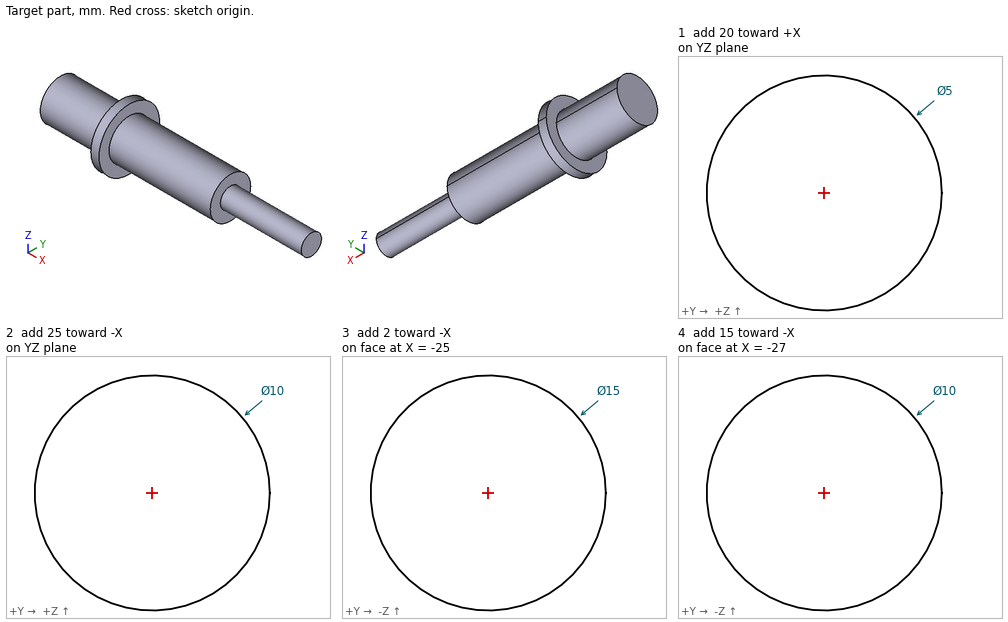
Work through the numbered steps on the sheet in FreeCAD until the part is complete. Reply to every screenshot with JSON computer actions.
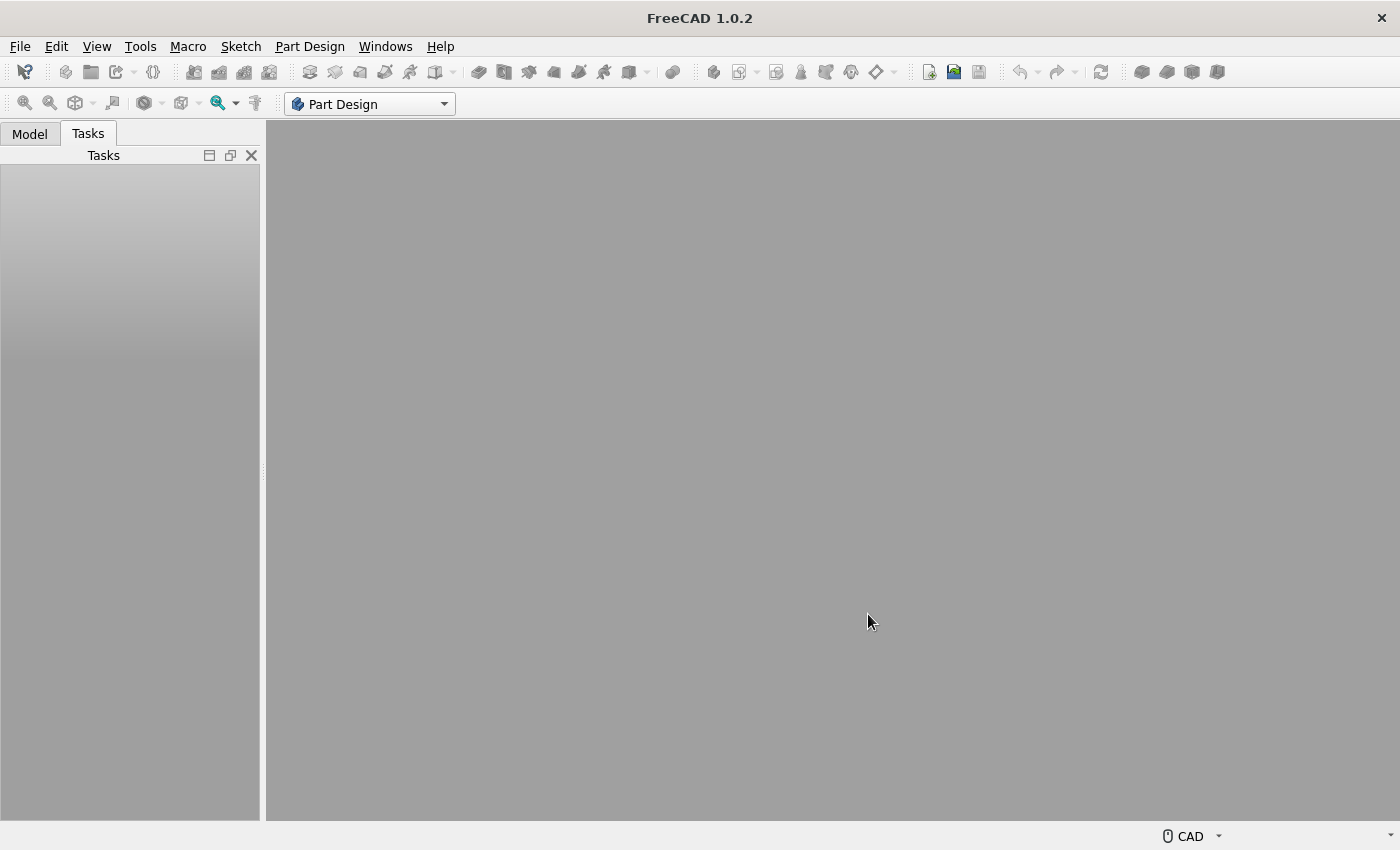
{"action": "key", "text": "ctrl+n"}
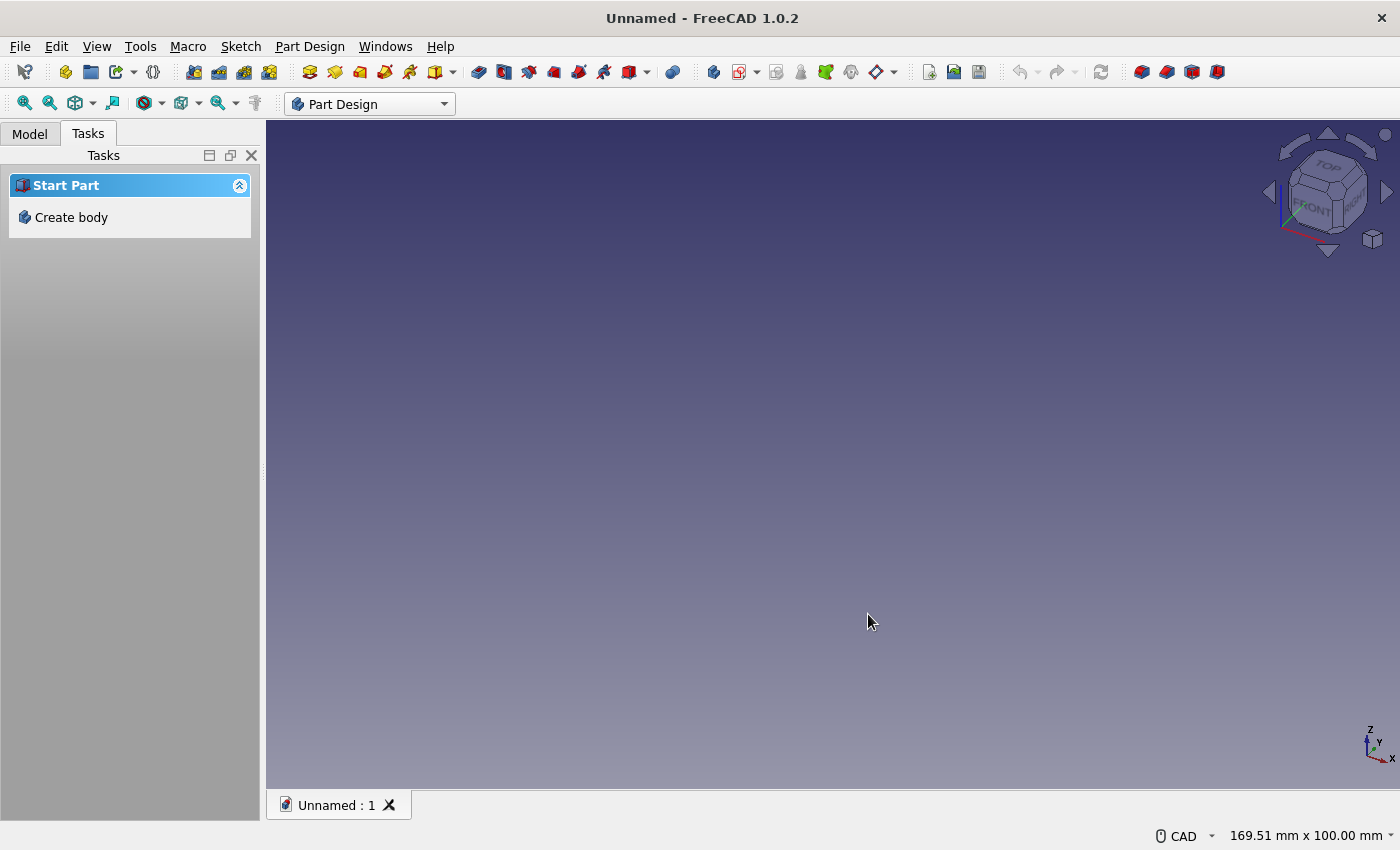
{"action": "left_click", "coordinate": [738, 72]}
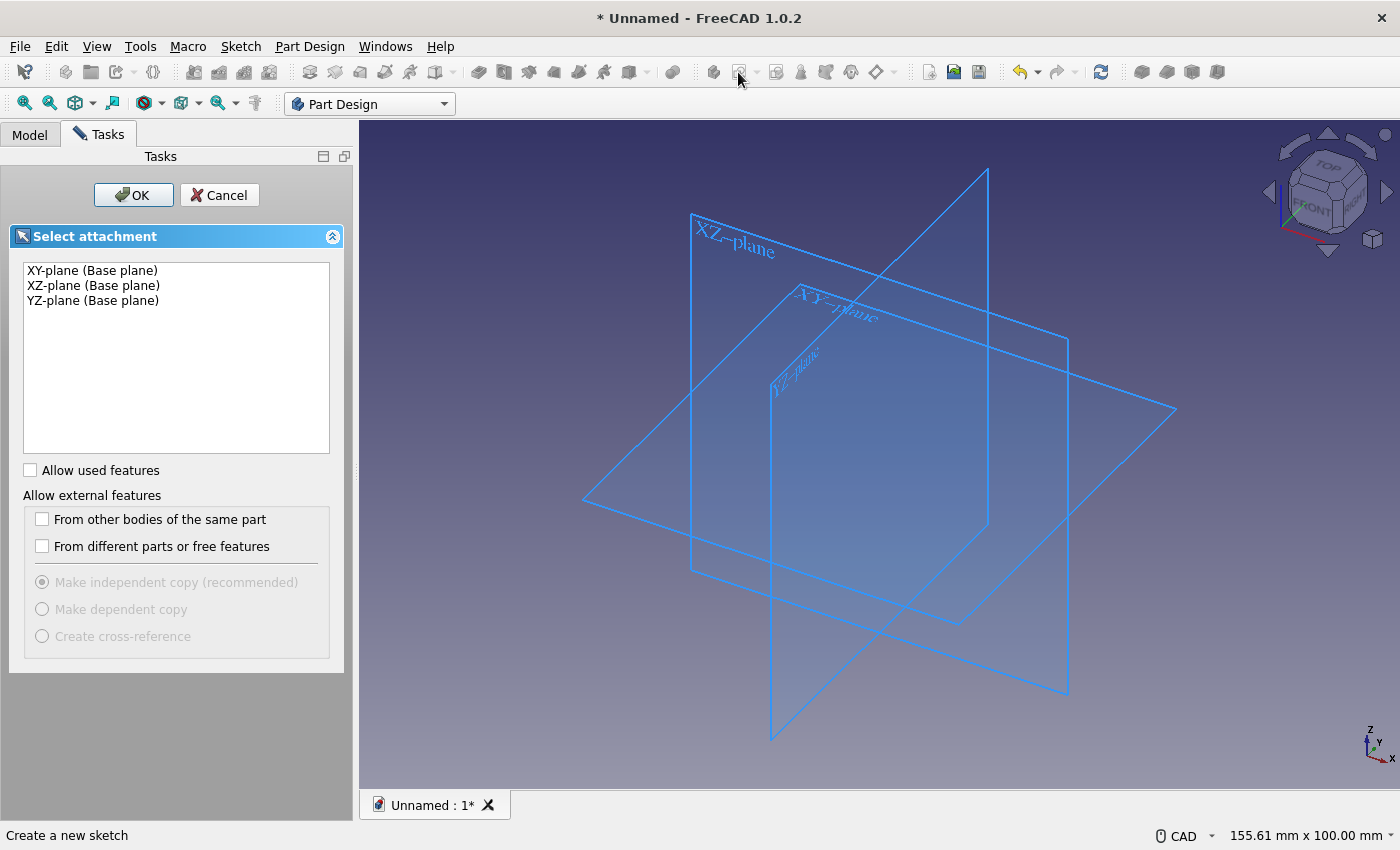
{"action": "left_click", "coordinate": [84, 300]}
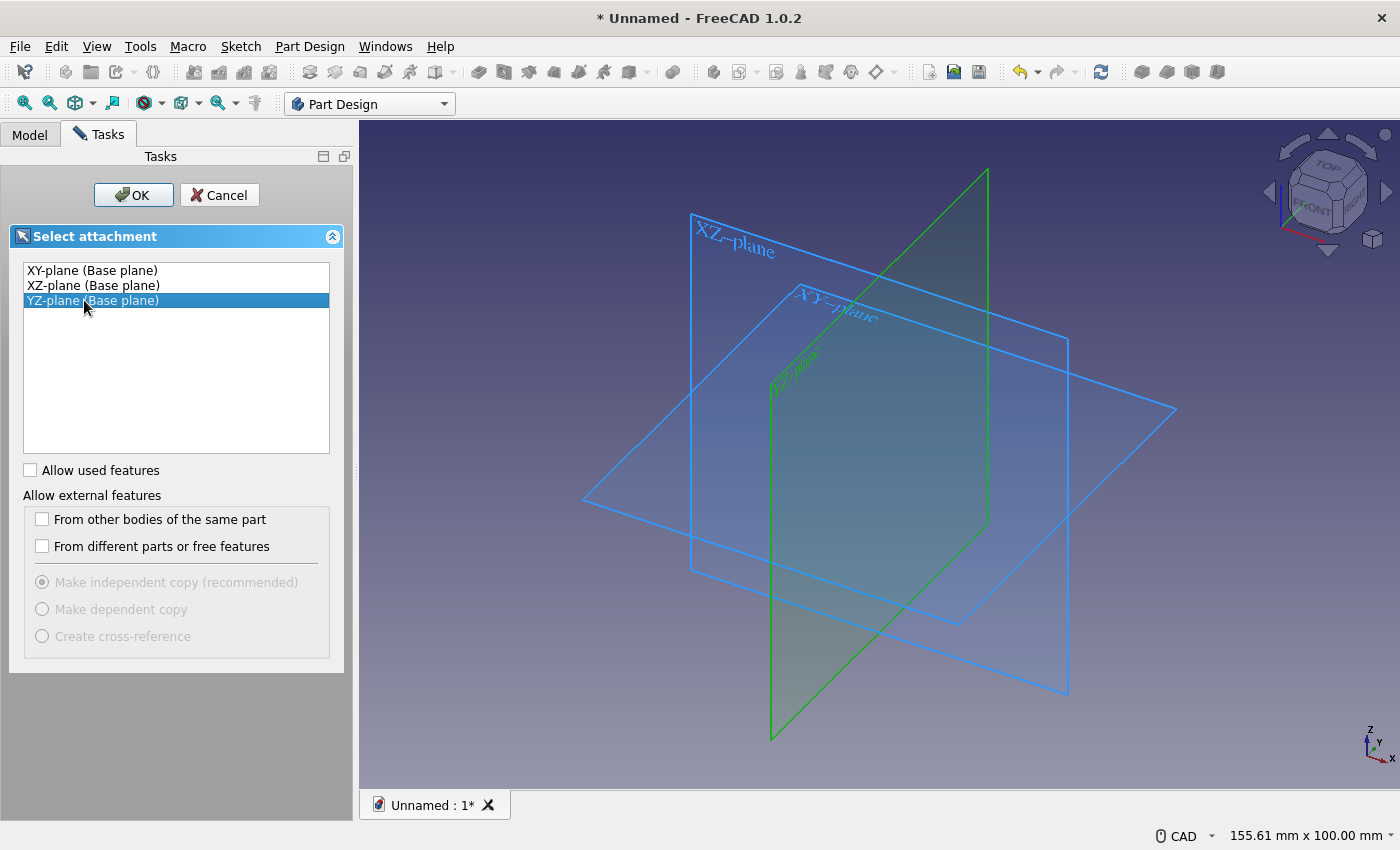
{"action": "left_click", "coordinate": [134, 195]}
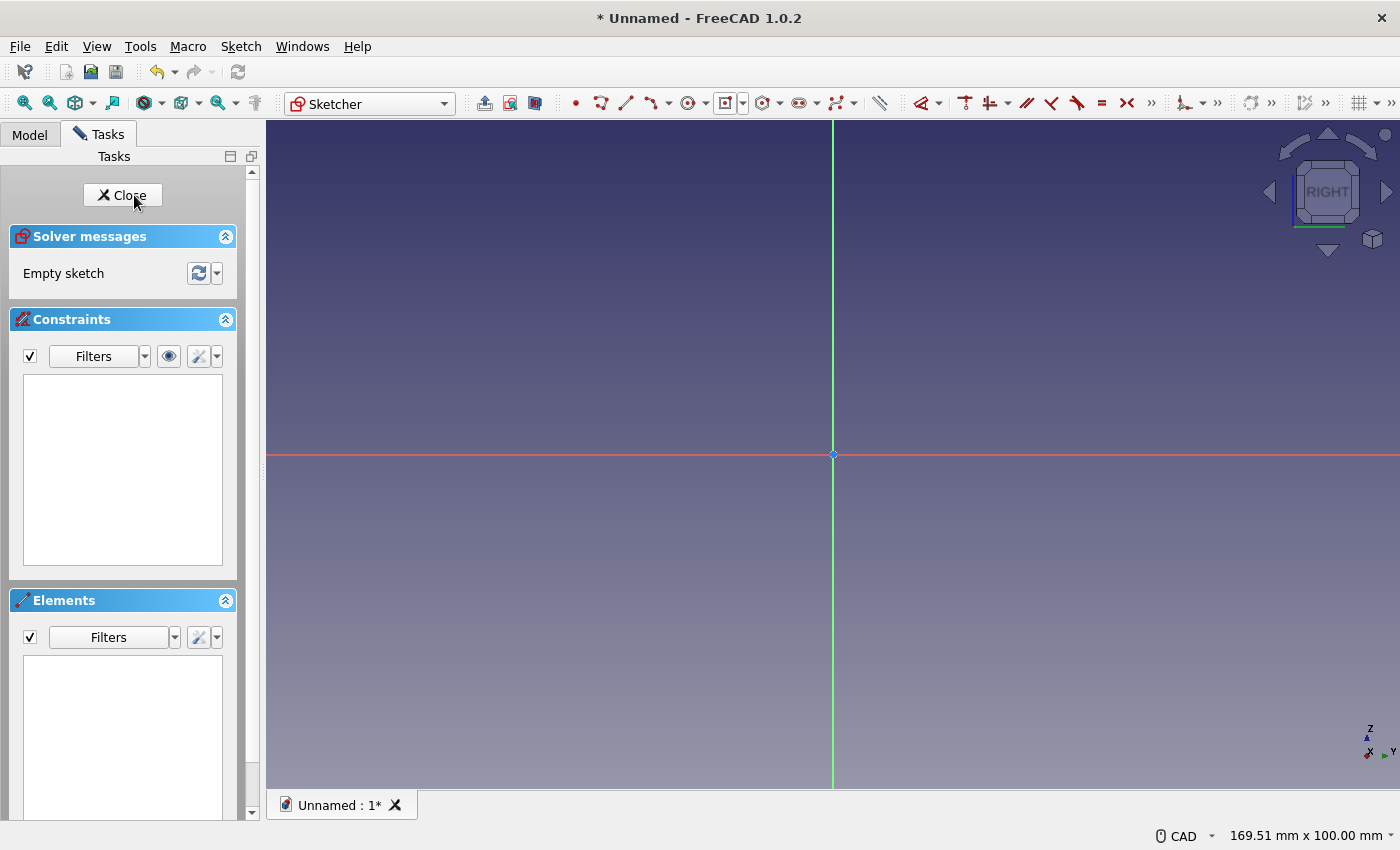
{"action": "scroll", "coordinate": [838, 454], "scroll_direction": "up", "scroll_amount": 13}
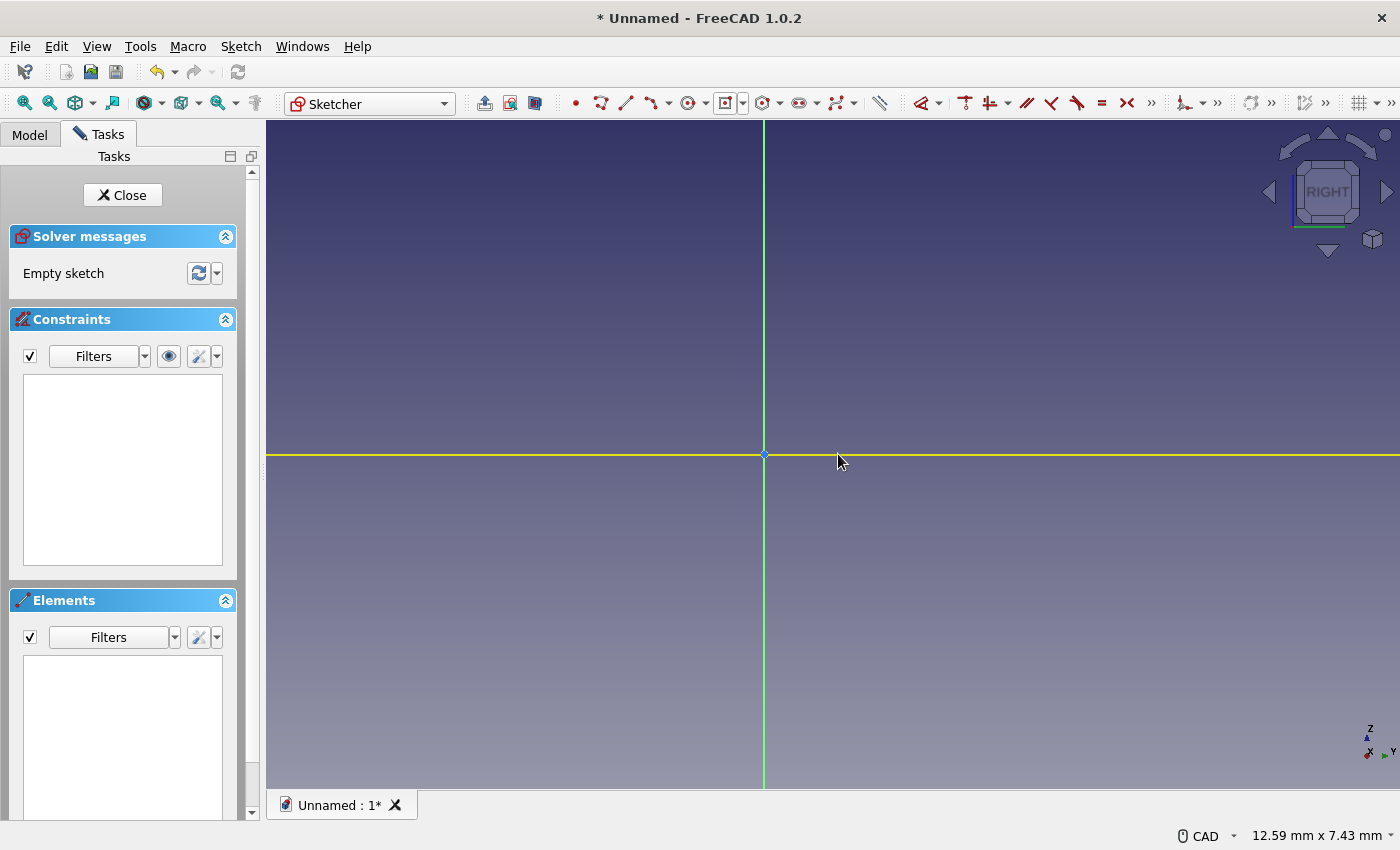
{"action": "key", "text": "g c"}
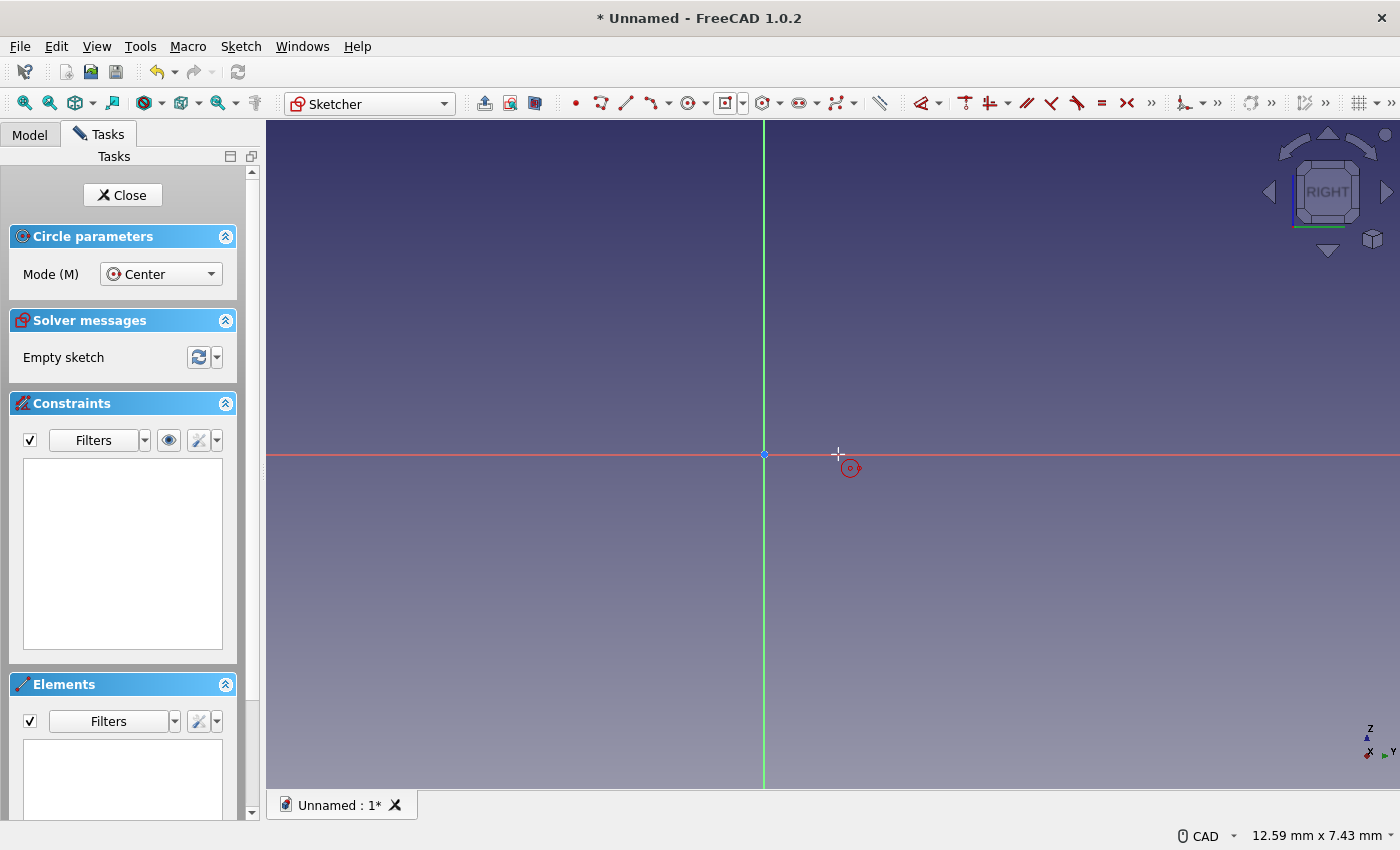
{"action": "left_click", "coordinate": [764, 454]}
{"action": "left_click", "coordinate": [924, 295]}
{"action": "key", "text": "Escape"}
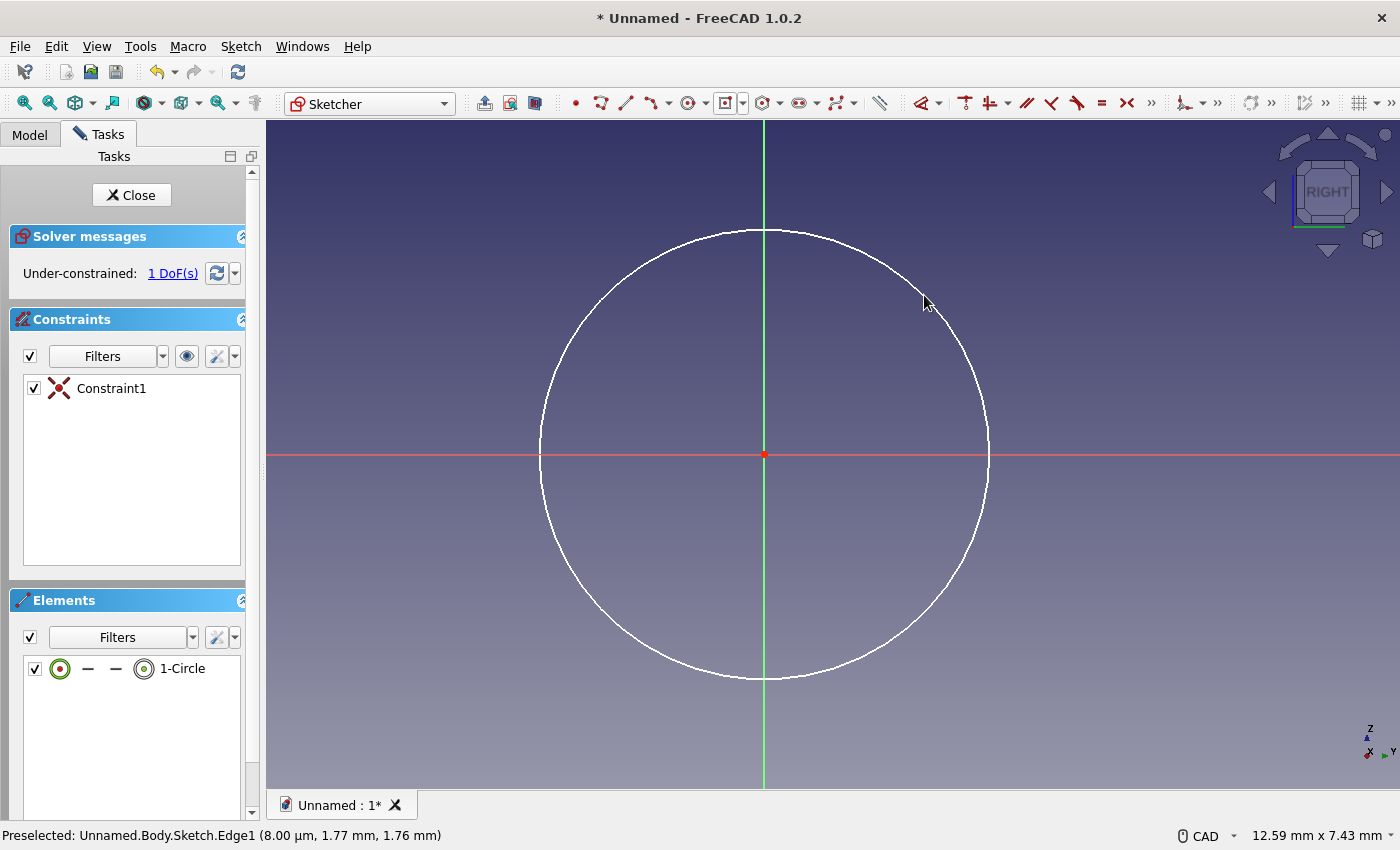
{"action": "key", "text": "d"}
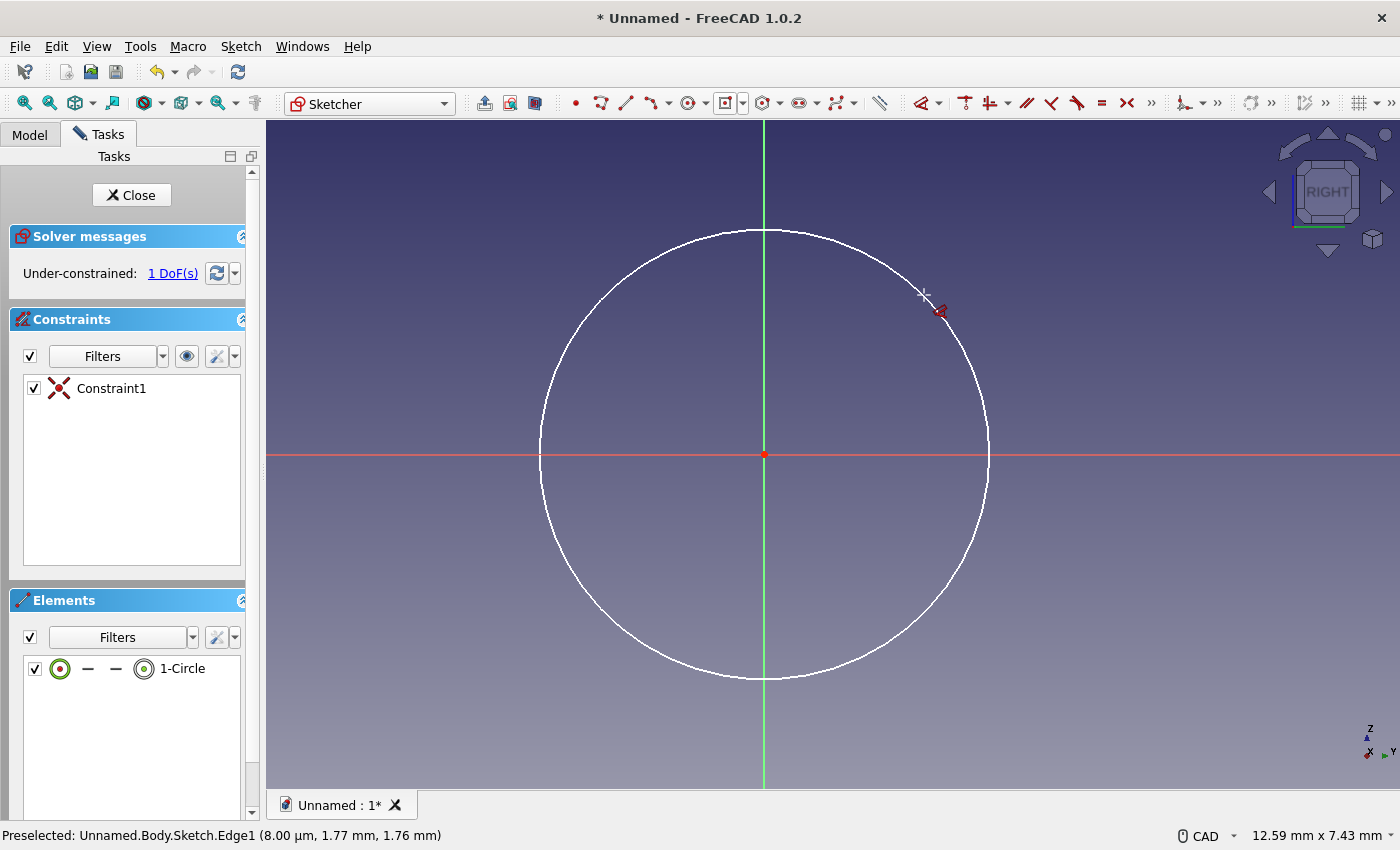
{"action": "left_click", "coordinate": [923, 295]}
{"action": "left_click", "coordinate": [946, 272]}